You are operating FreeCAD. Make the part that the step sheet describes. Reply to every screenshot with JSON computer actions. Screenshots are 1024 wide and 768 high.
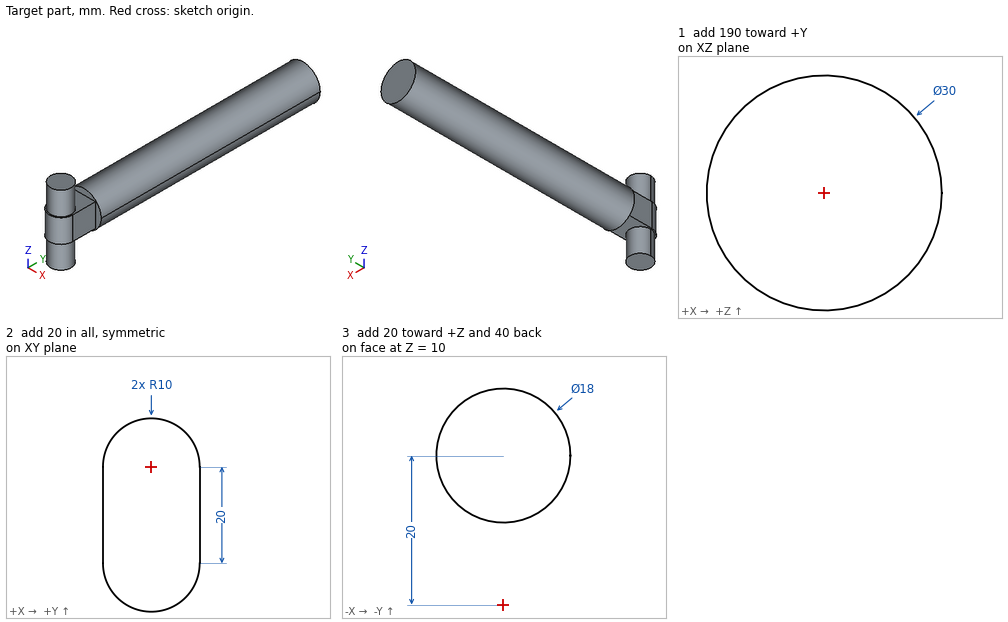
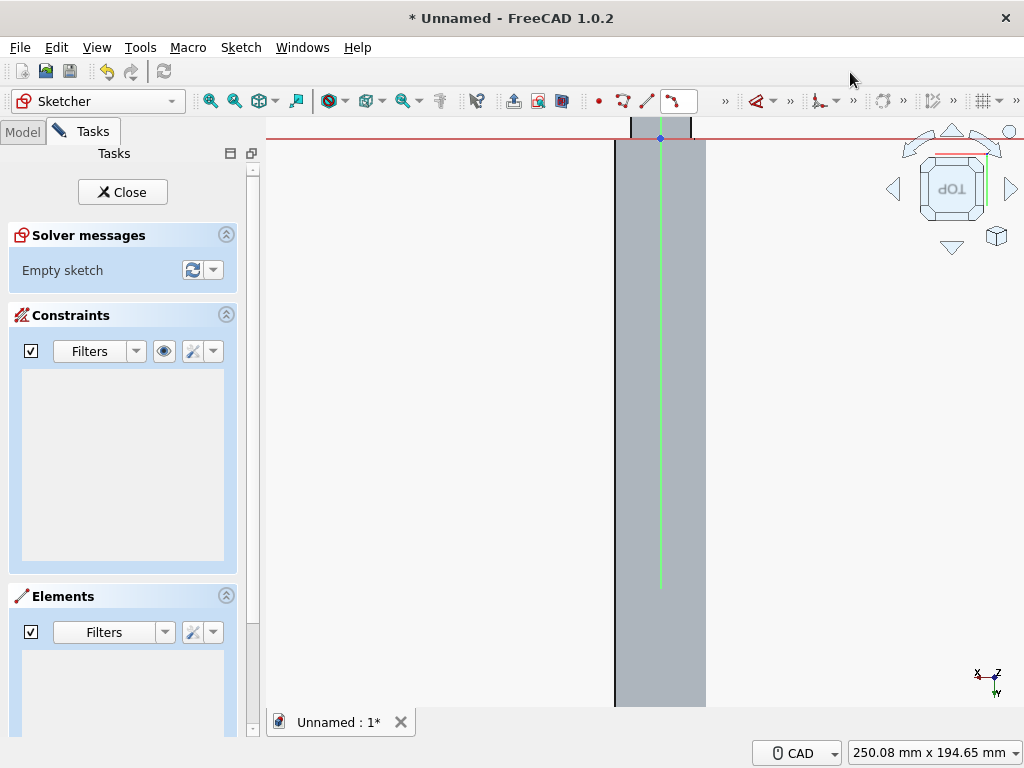
{"action": "scroll", "coordinate": [576, 412], "scroll_direction": "down", "scroll_amount": 5}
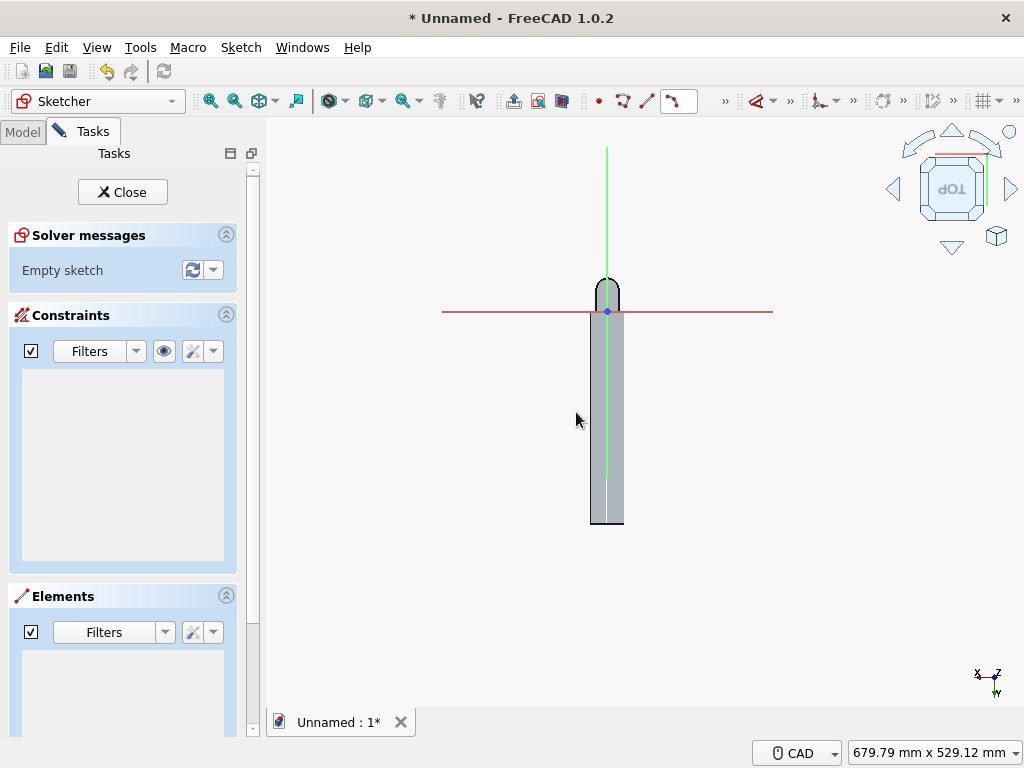
{"action": "scroll", "coordinate": [611, 284], "scroll_direction": "up", "scroll_amount": 12}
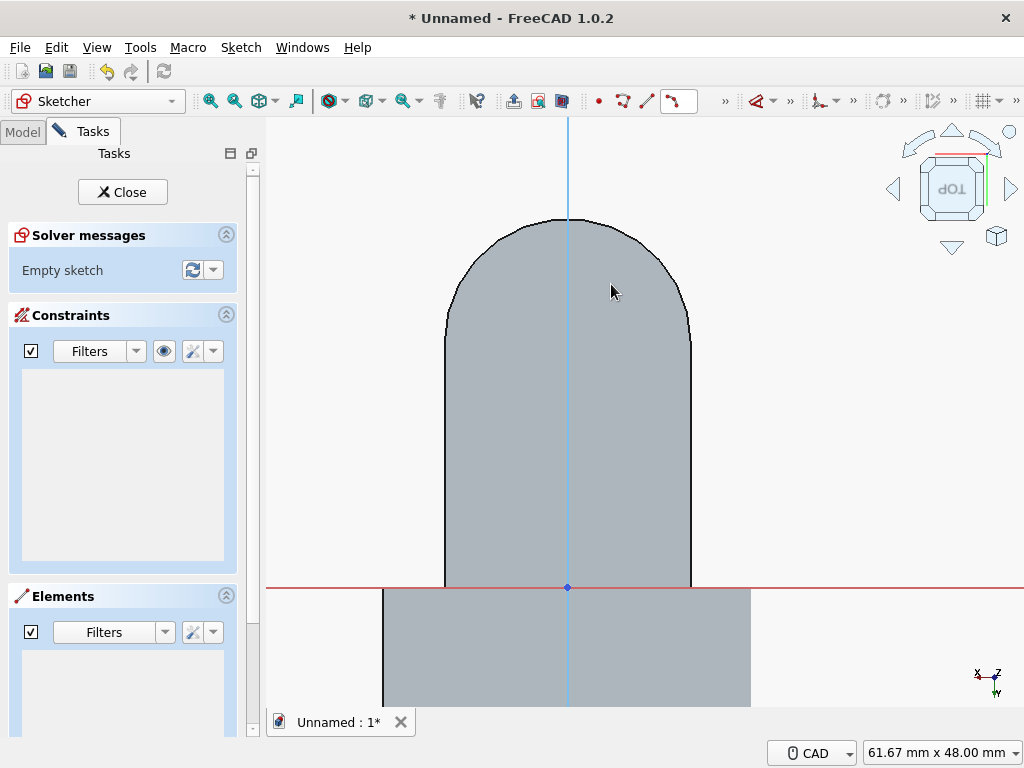
{"action": "key", "text": "g c"}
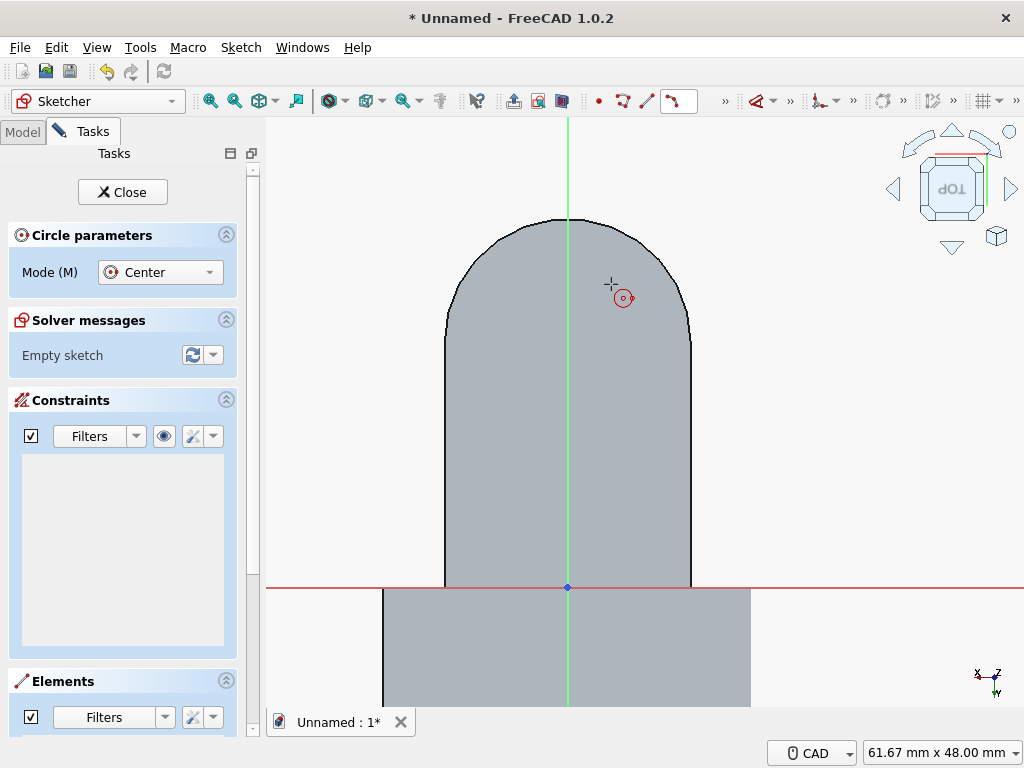
{"action": "left_click", "coordinate": [568, 342]}
{"action": "mouse_move", "coordinate": [646, 264]}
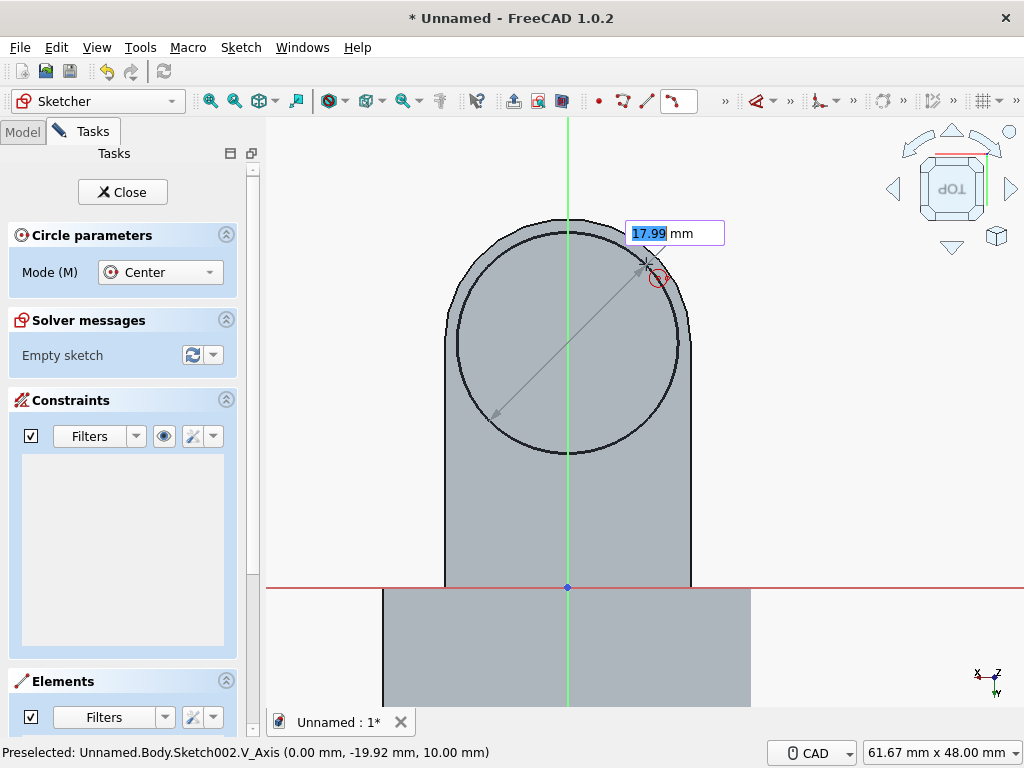
{"action": "type", "text": "18"}
{"action": "key", "text": "Return"}
{"action": "key", "text": "Escape"}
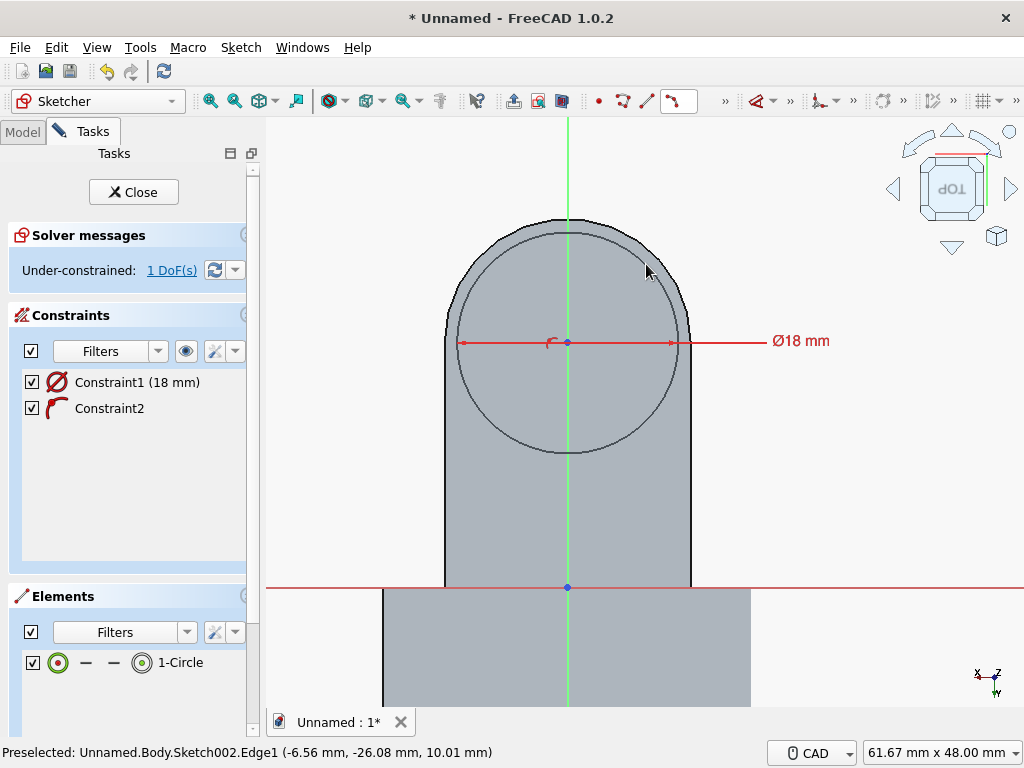
{"action": "key", "text": "d"}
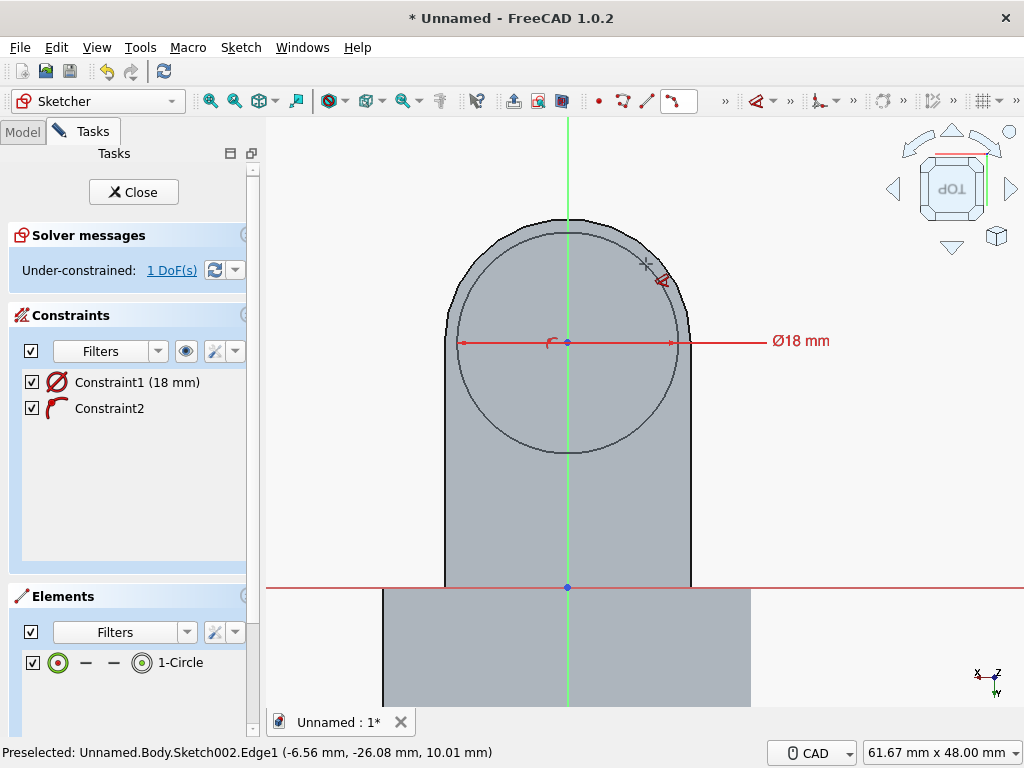
{"action": "left_click", "coordinate": [568, 343]}
{"action": "left_click", "coordinate": [602, 465]}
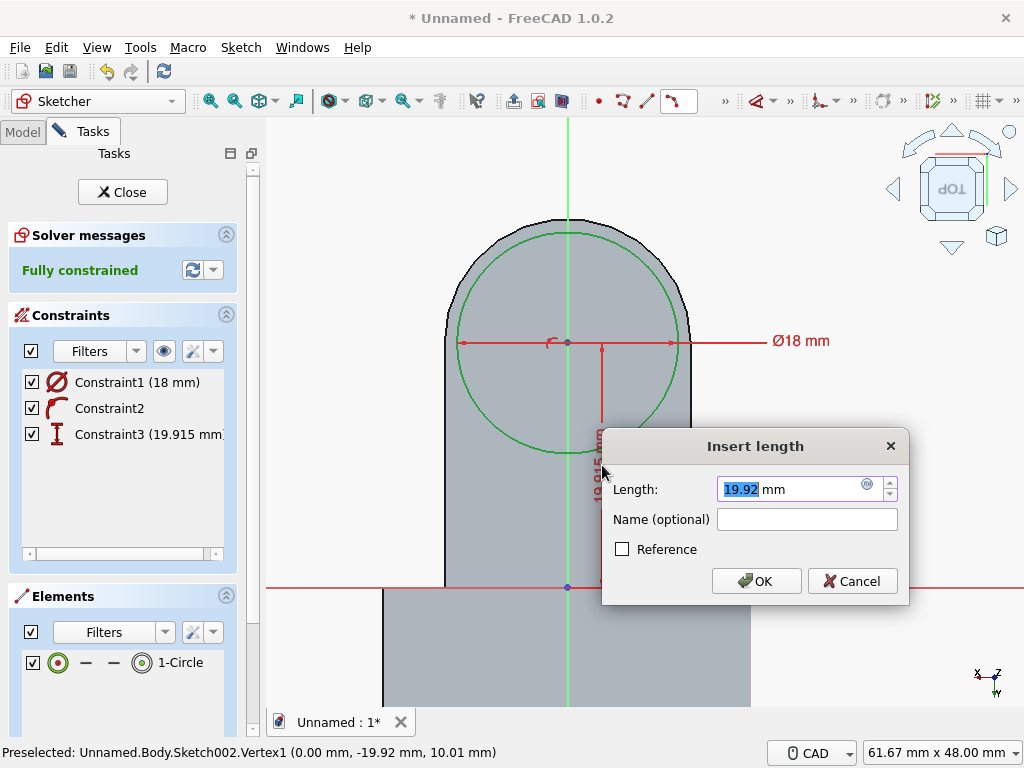
{"action": "type", "text": "20"}
{"action": "key", "text": "Return"}
{"action": "key", "text": "Escape"}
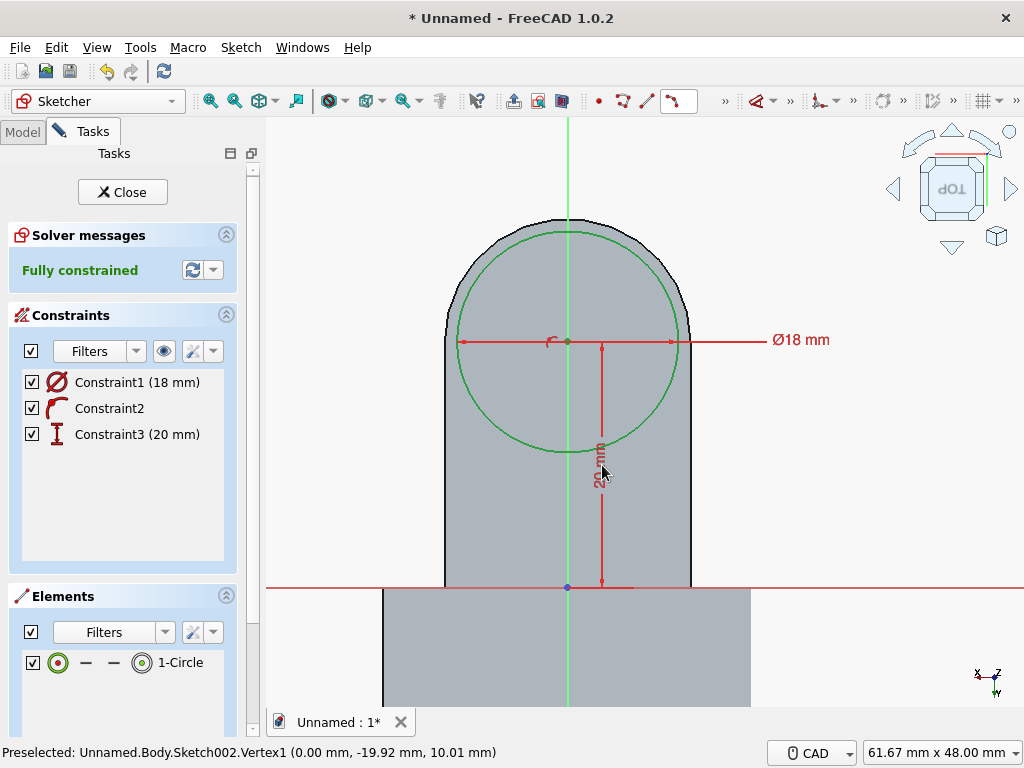
{"action": "left_click", "coordinate": [123, 192]}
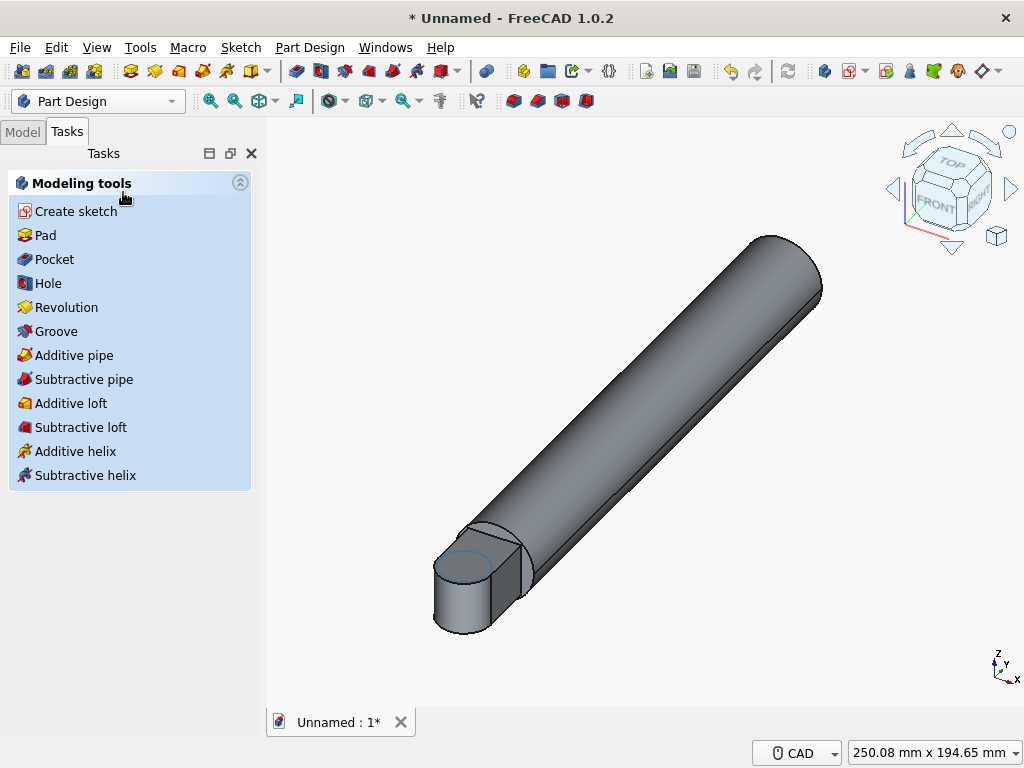
{"action": "left_click", "coordinate": [132, 72]}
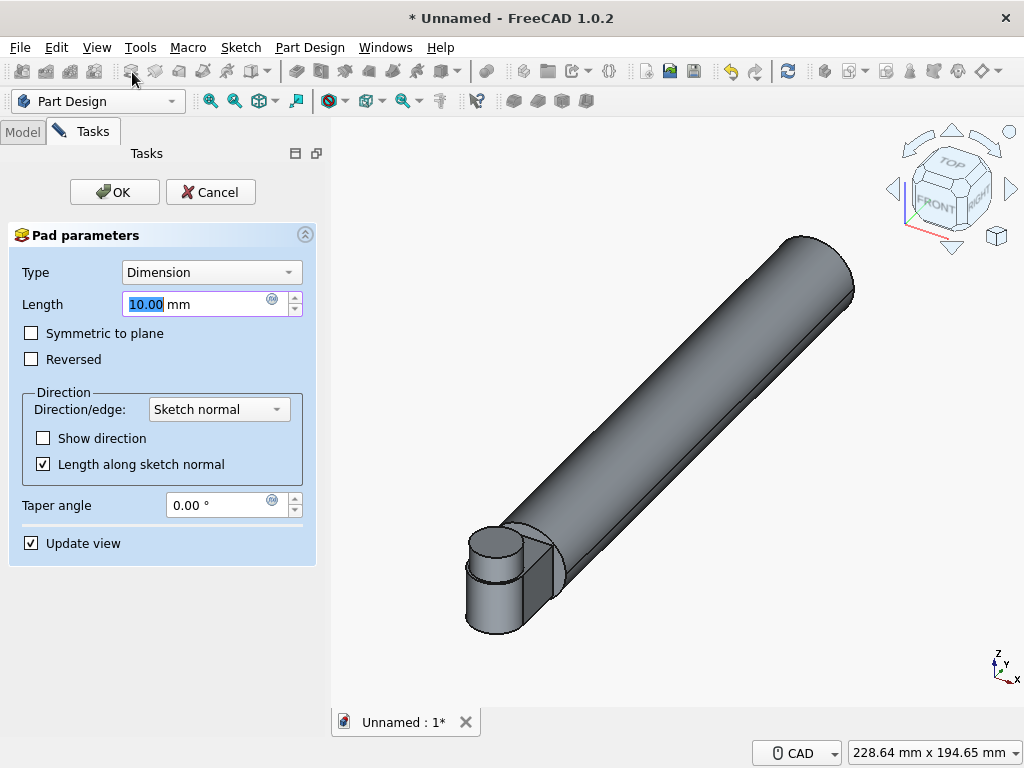
{"action": "left_click", "coordinate": [212, 272]}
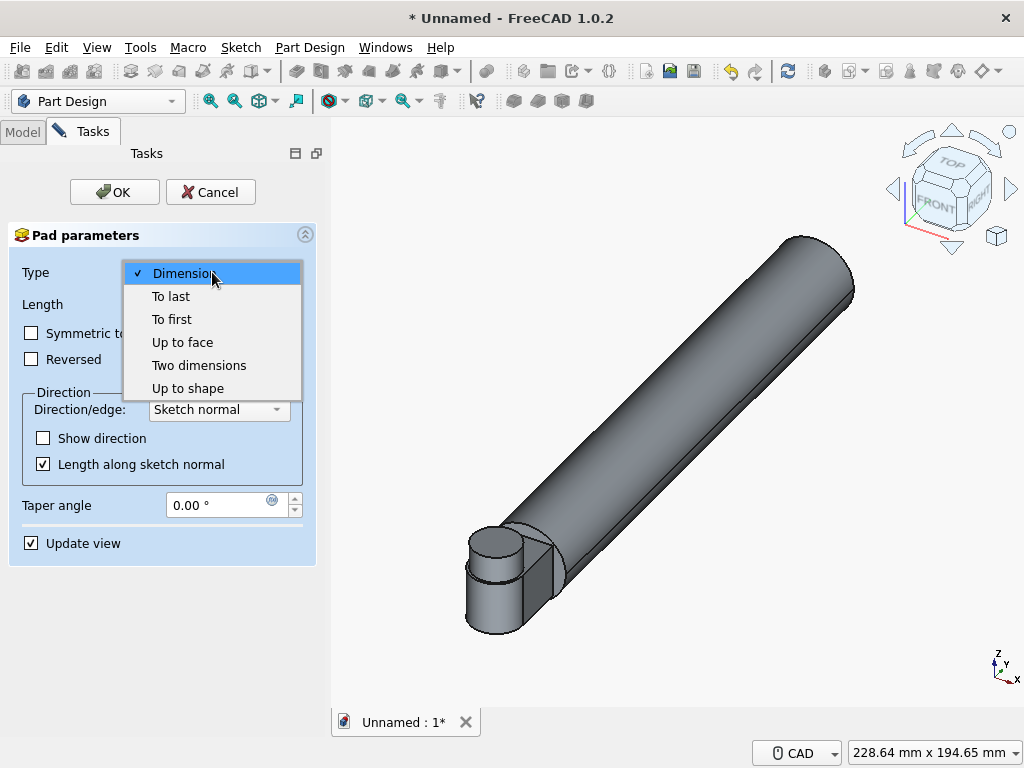
{"action": "left_click", "coordinate": [212, 366]}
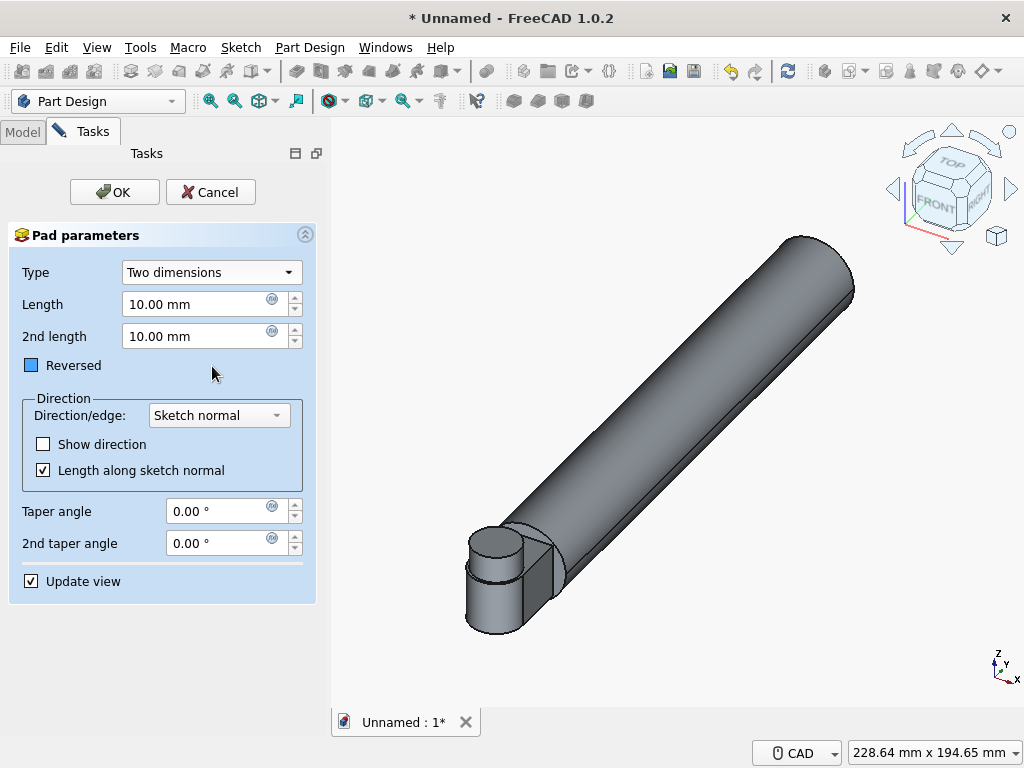
{"action": "triple_click", "coordinate": [204, 304]}